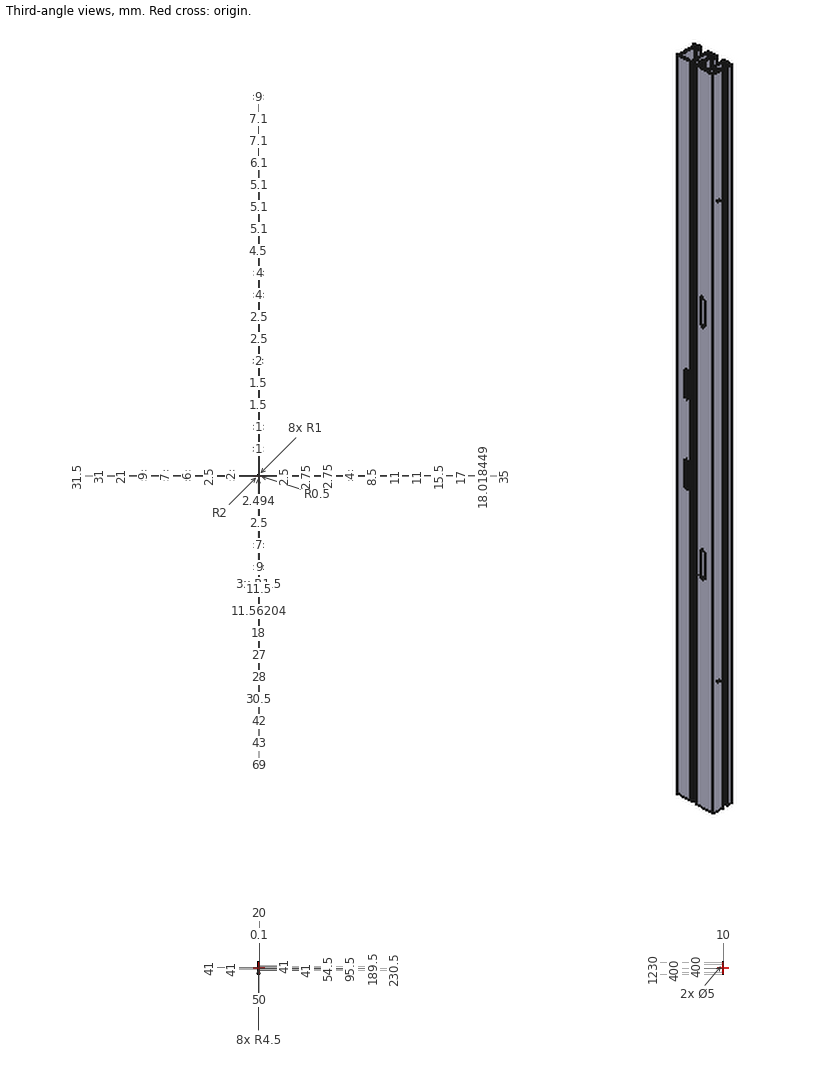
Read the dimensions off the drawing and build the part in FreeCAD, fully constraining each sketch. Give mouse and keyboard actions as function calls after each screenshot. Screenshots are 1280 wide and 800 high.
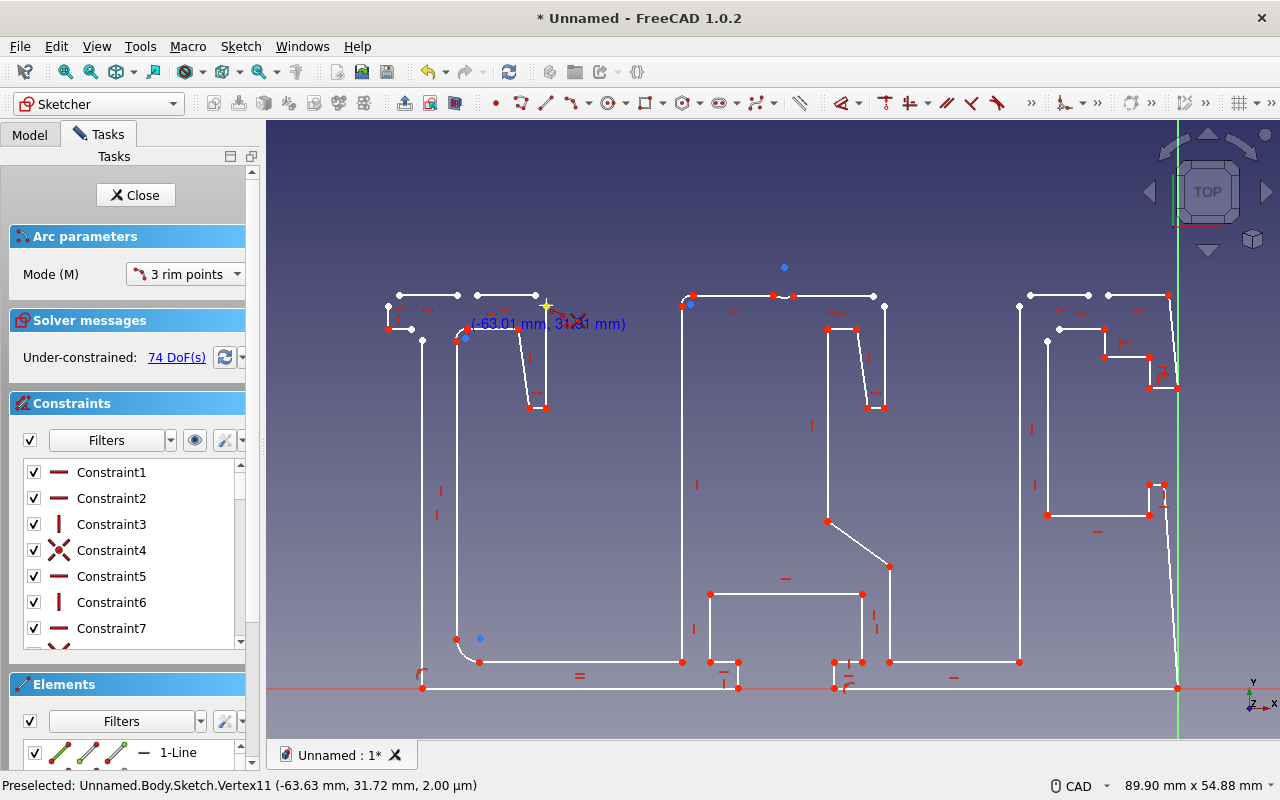
click(546, 306)
click(535, 295)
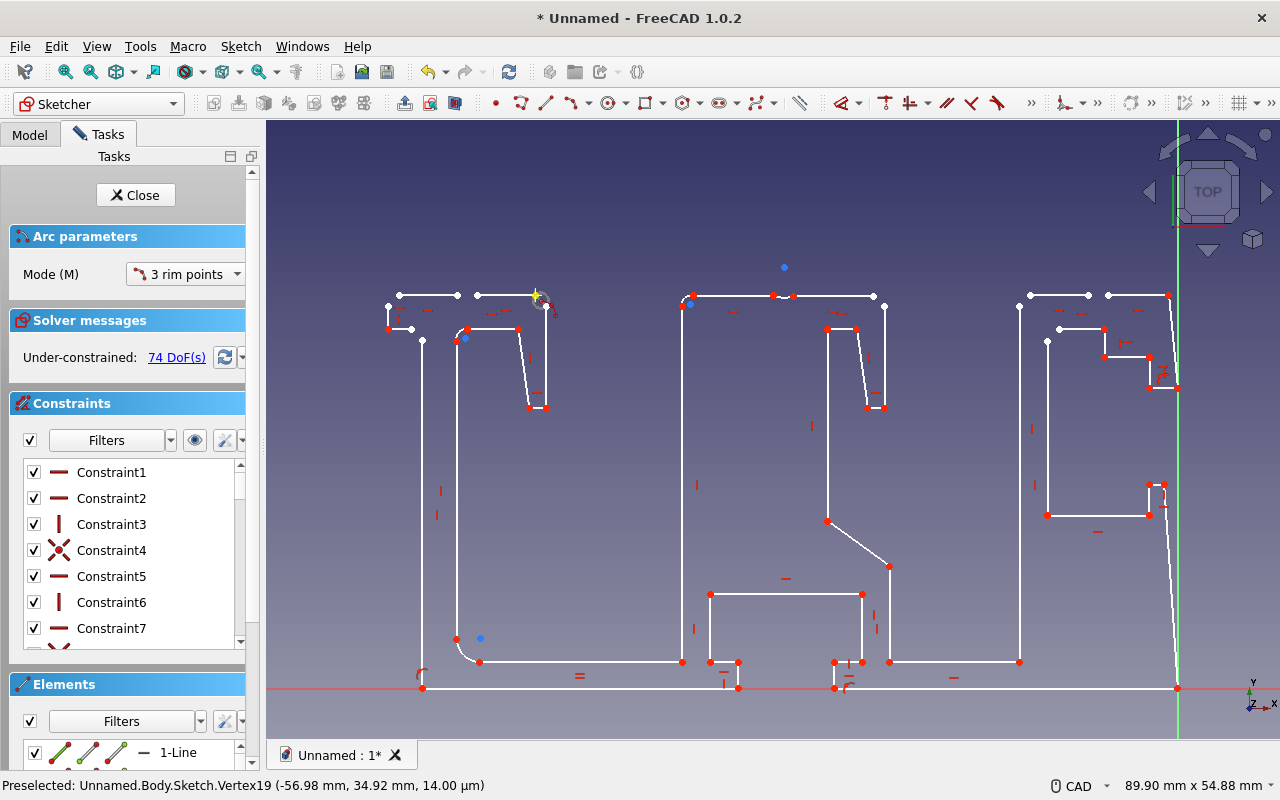
scroll(543, 297, up, 8)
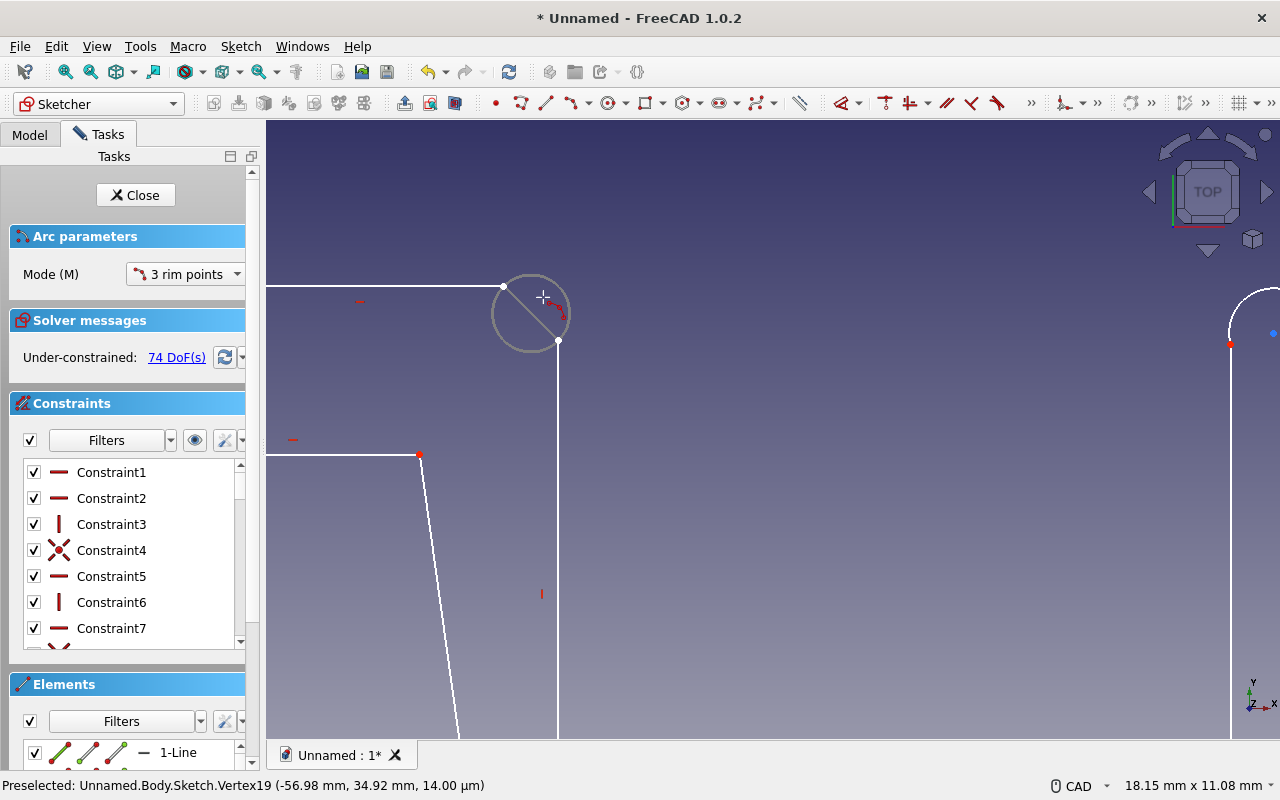
click(542, 298)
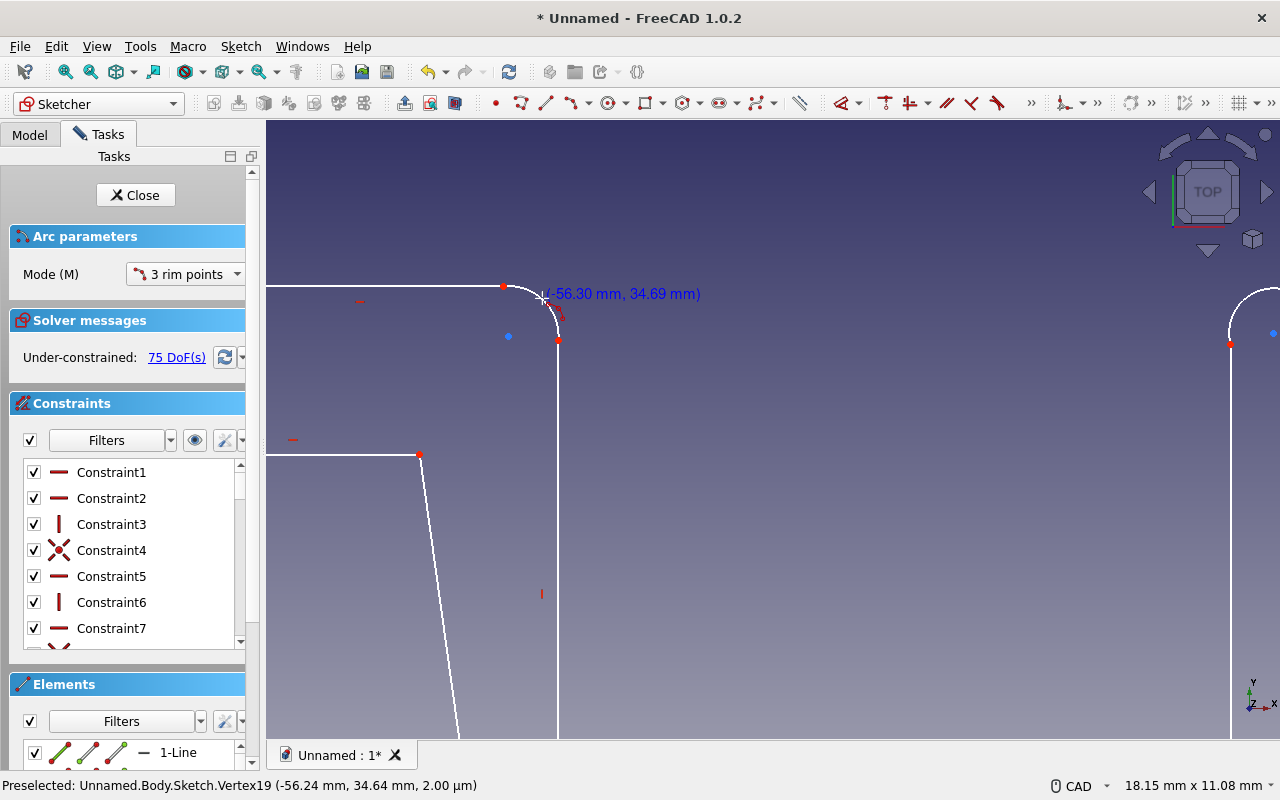
scroll(544, 300, down, 10)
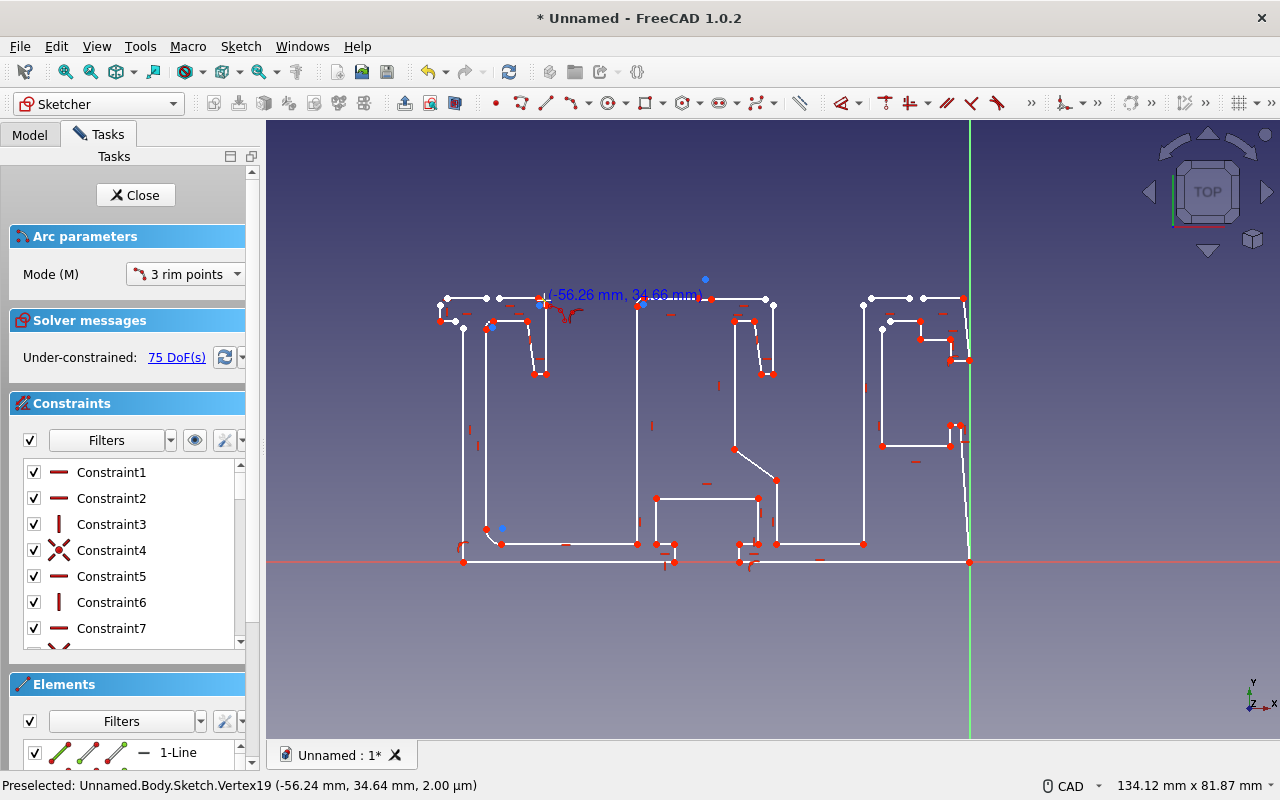
click(500, 298)
click(487, 298)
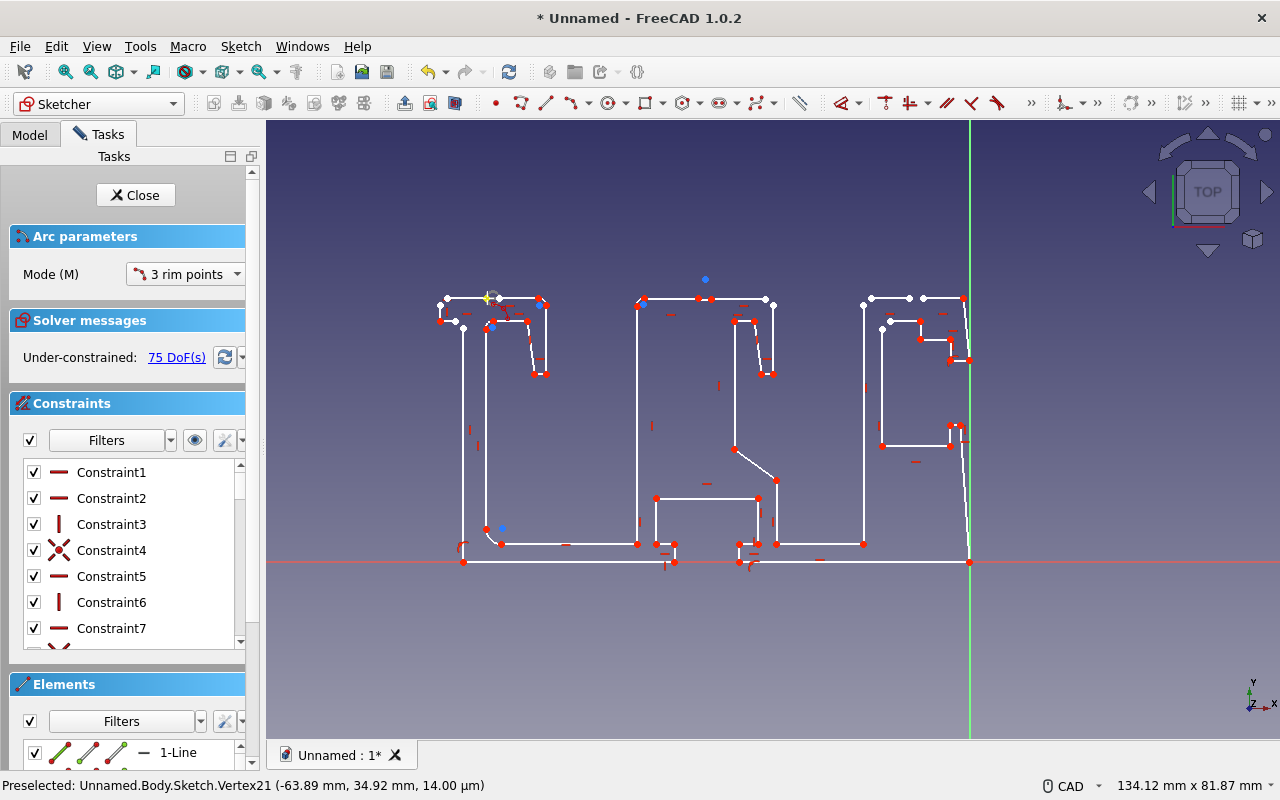
scroll(493, 300, up, 10)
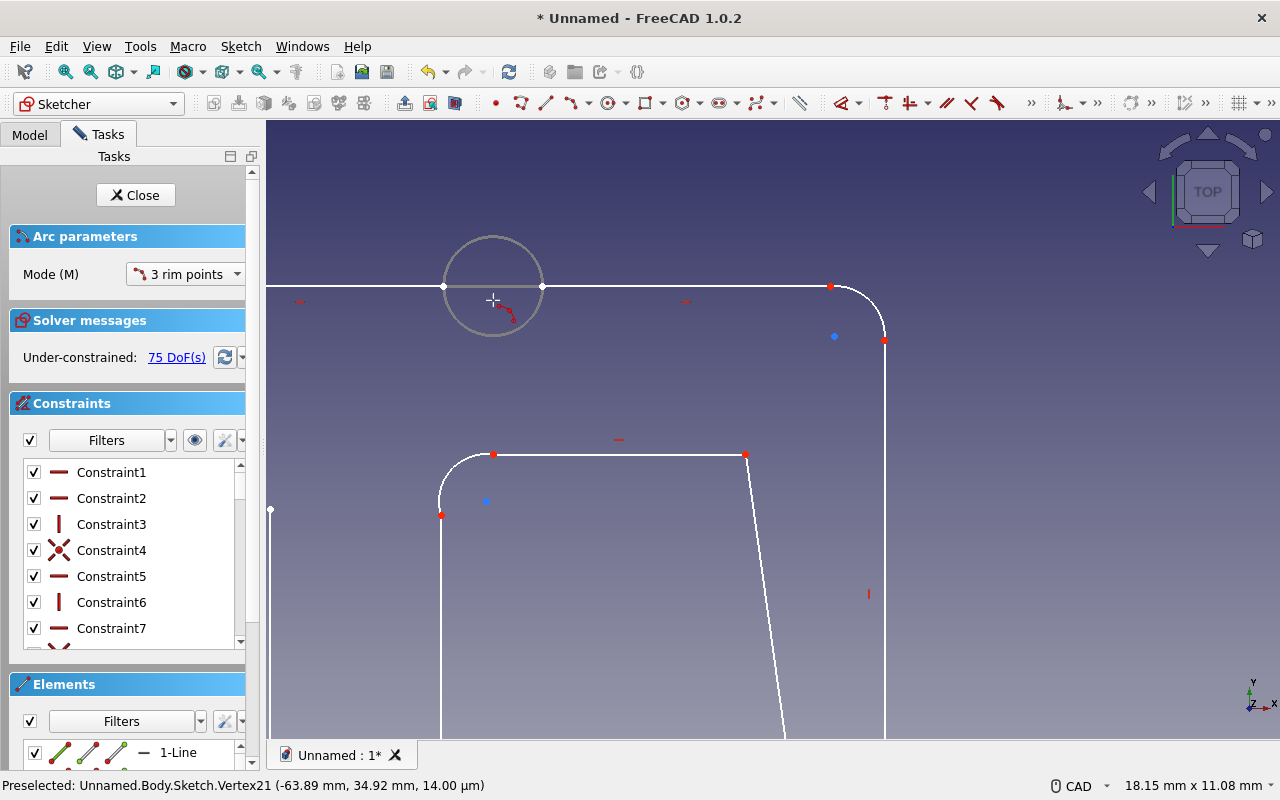
click(494, 299)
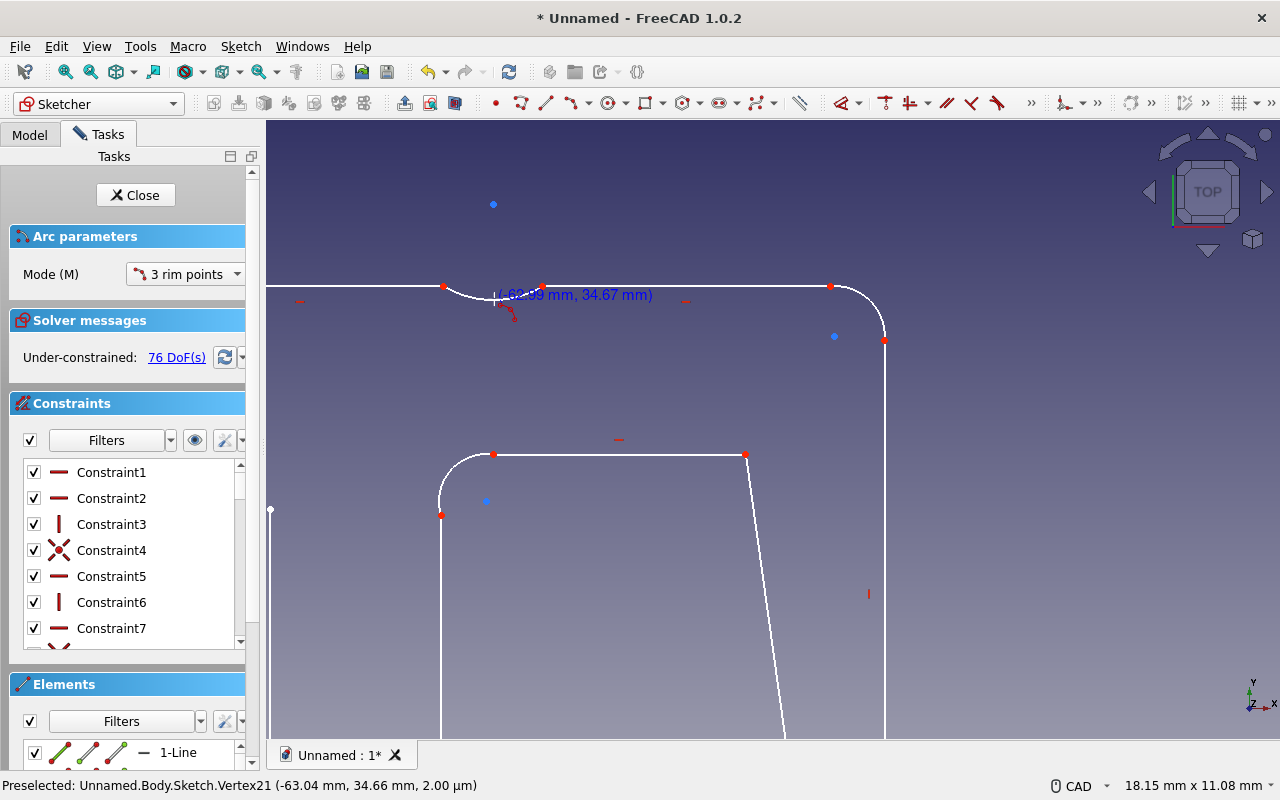
scroll(493, 300, down, 10)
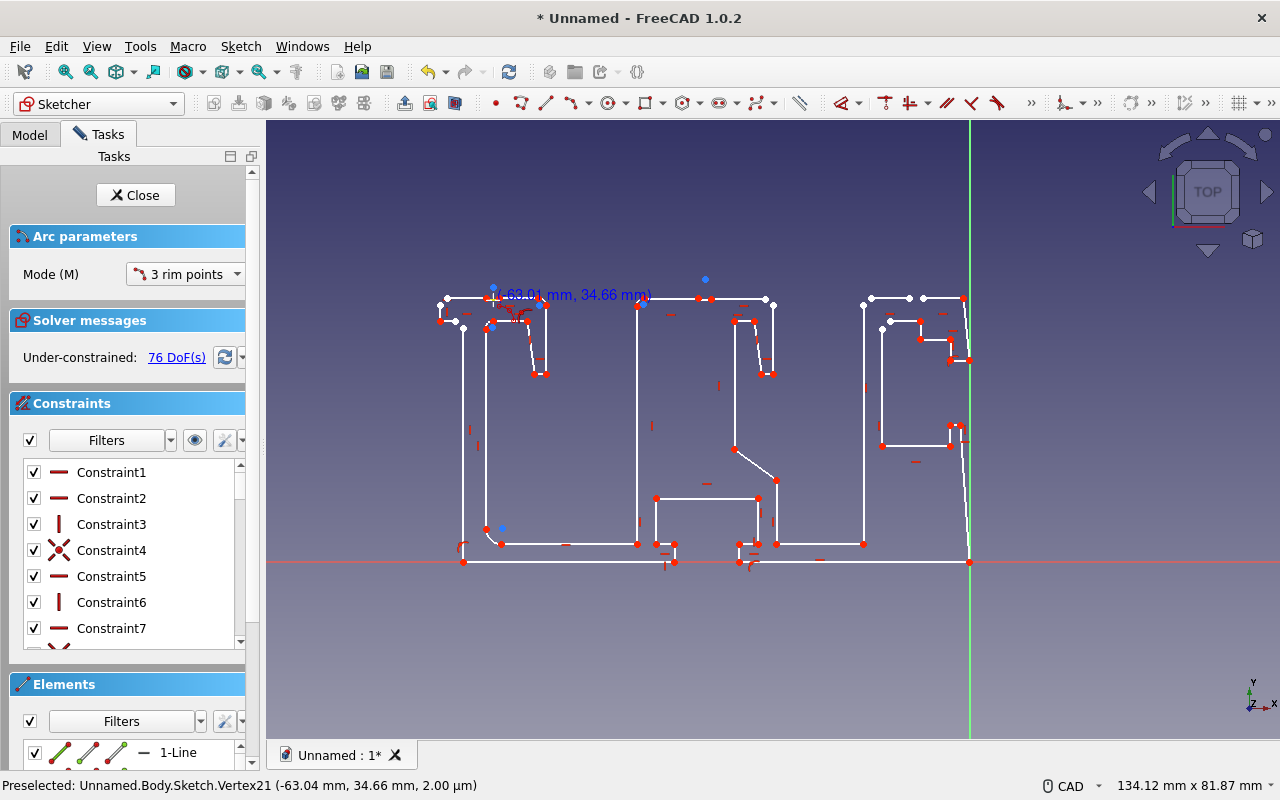
scroll(448, 298, up, 2)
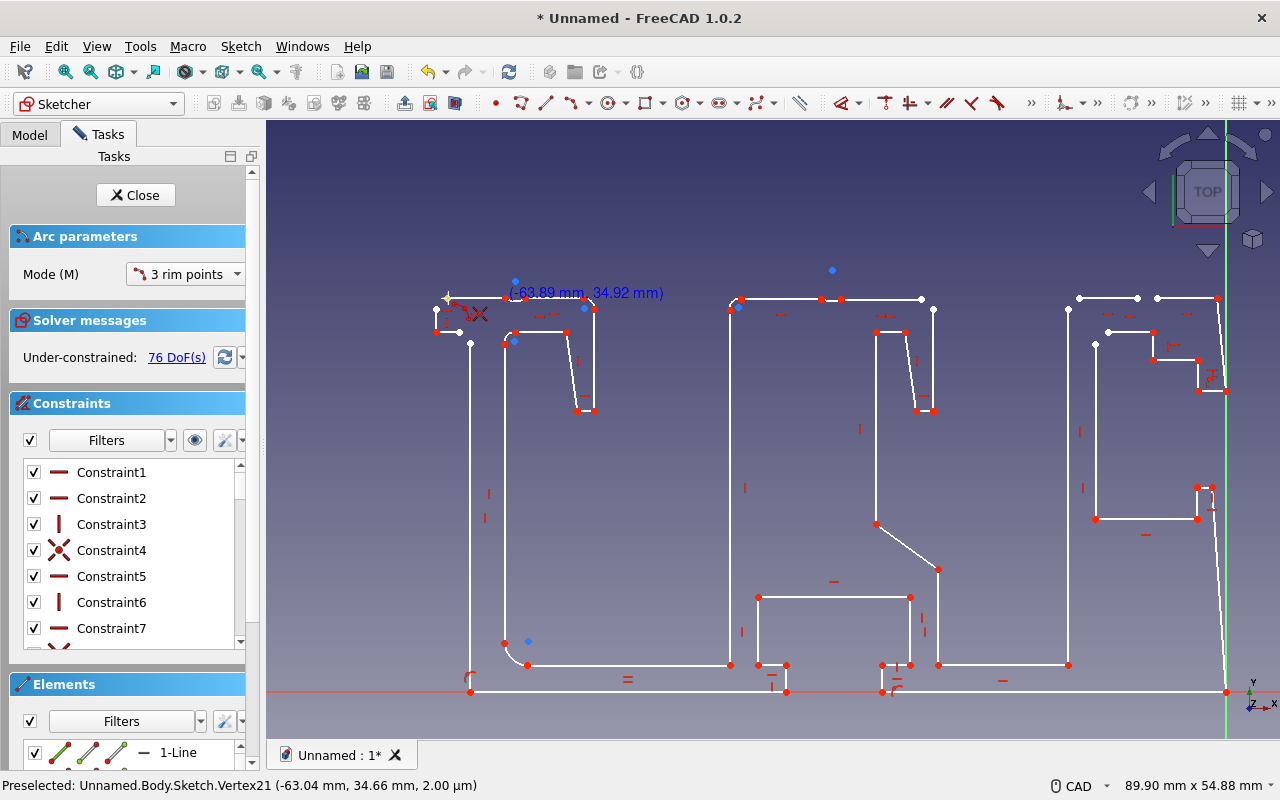
click(447, 298)